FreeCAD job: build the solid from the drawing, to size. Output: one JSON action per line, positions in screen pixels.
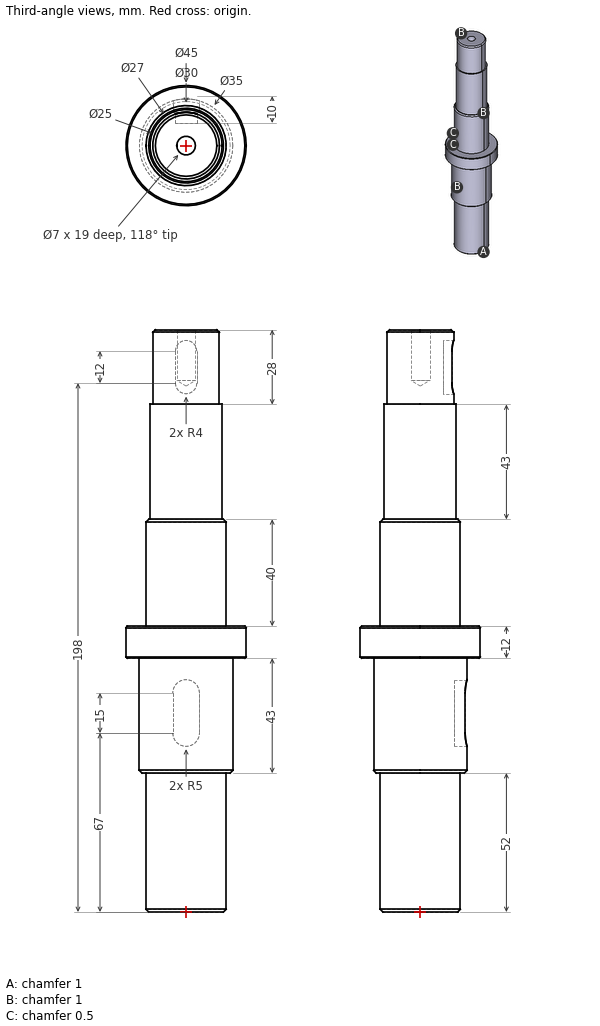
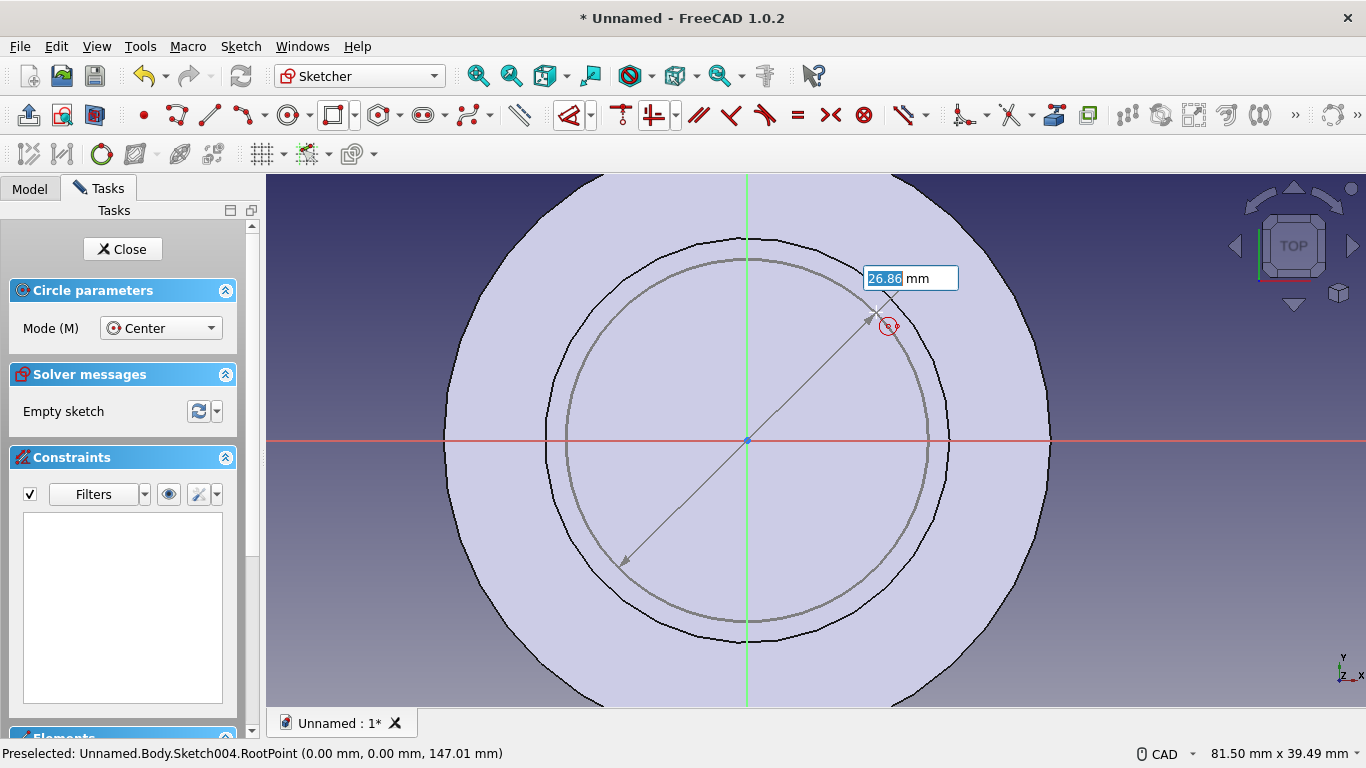
{"action": "type", "text": "27"}
{"action": "key", "text": "Return"}
{"action": "key", "text": "Escape"}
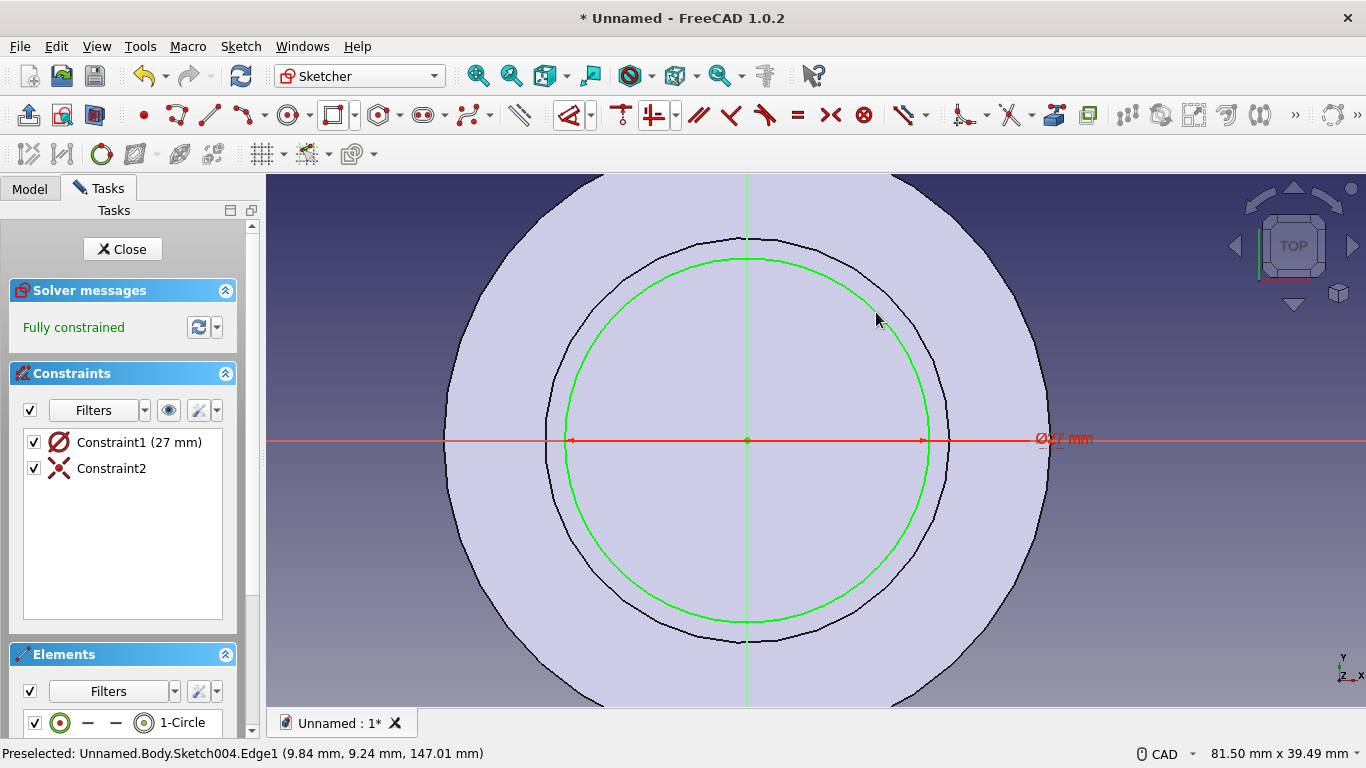
{"action": "left_click", "coordinate": [123, 249]}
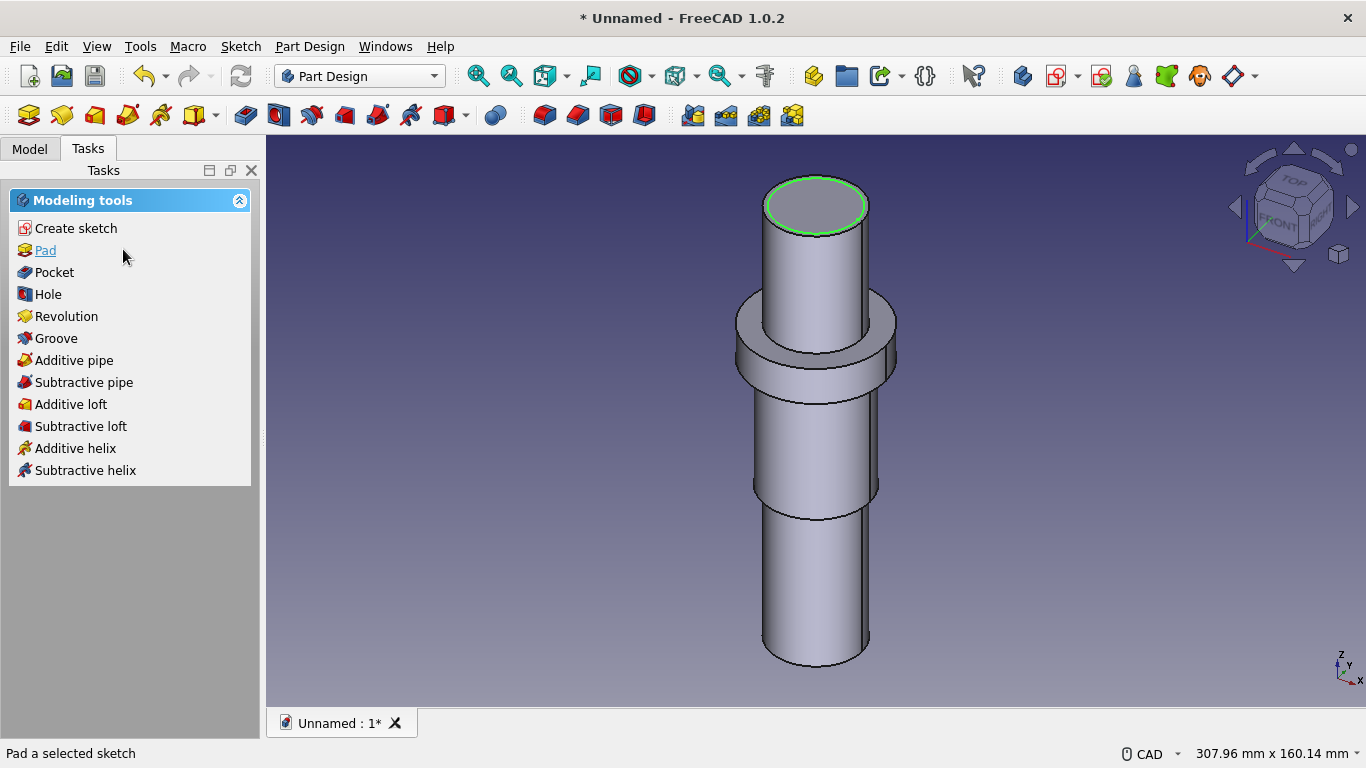
{"action": "left_click", "coordinate": [29, 116]}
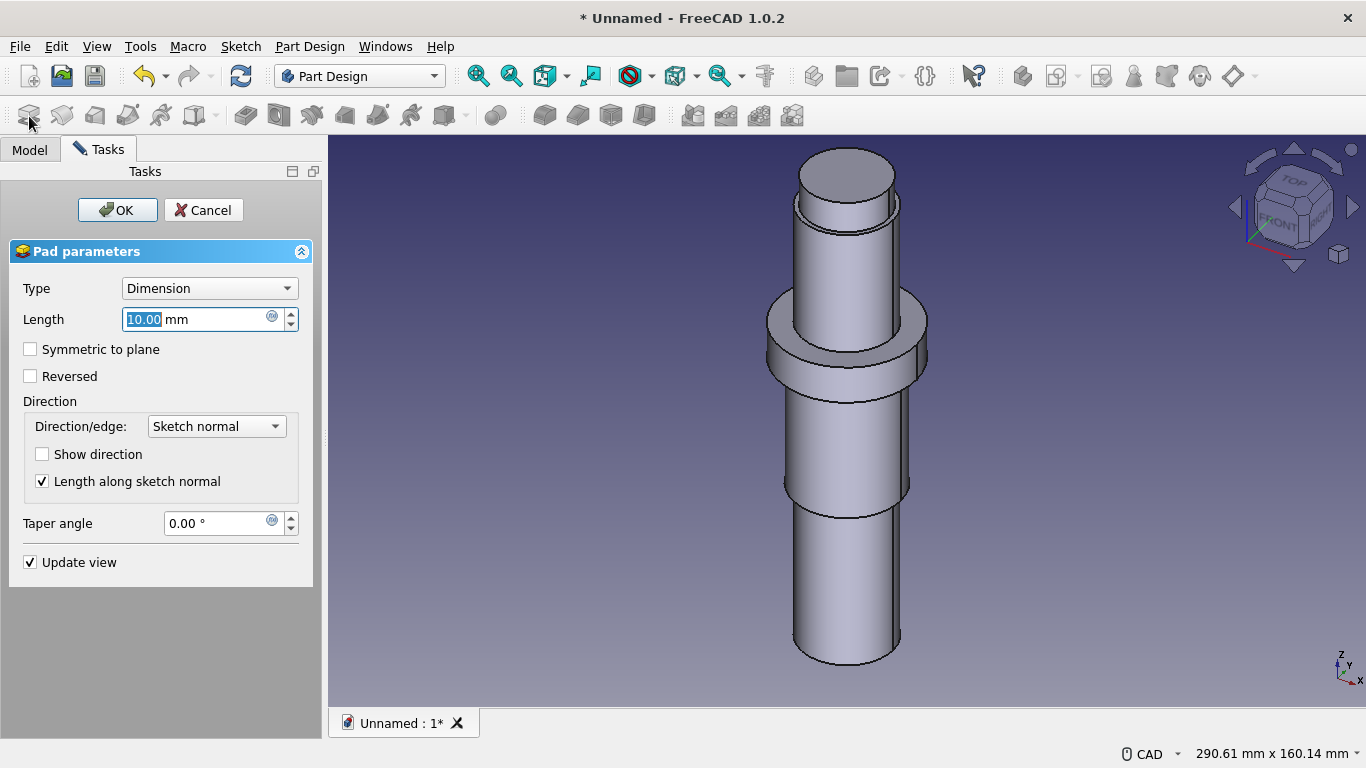
{"action": "type", "text": "43"}
{"action": "key", "text": "Tab"}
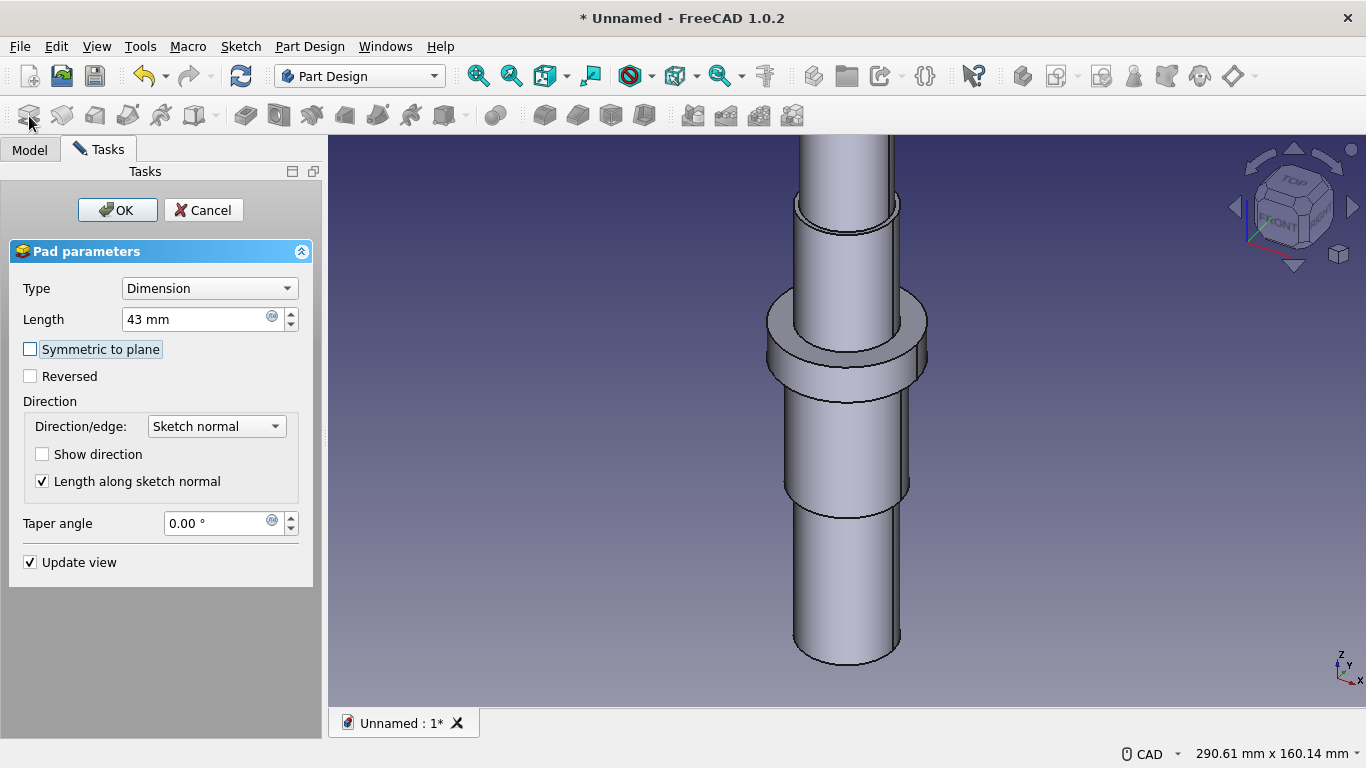
{"action": "left_click", "coordinate": [118, 210]}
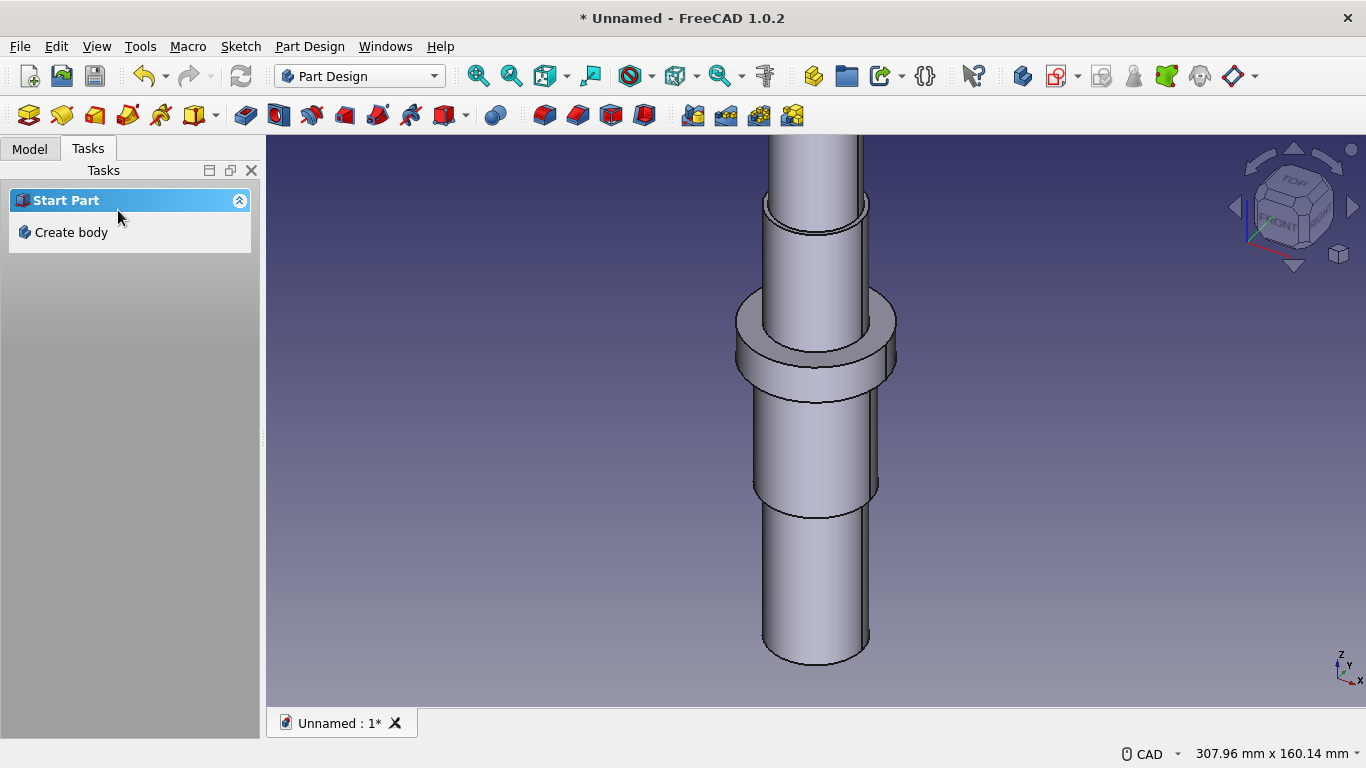
{"action": "key", "text": "v f"}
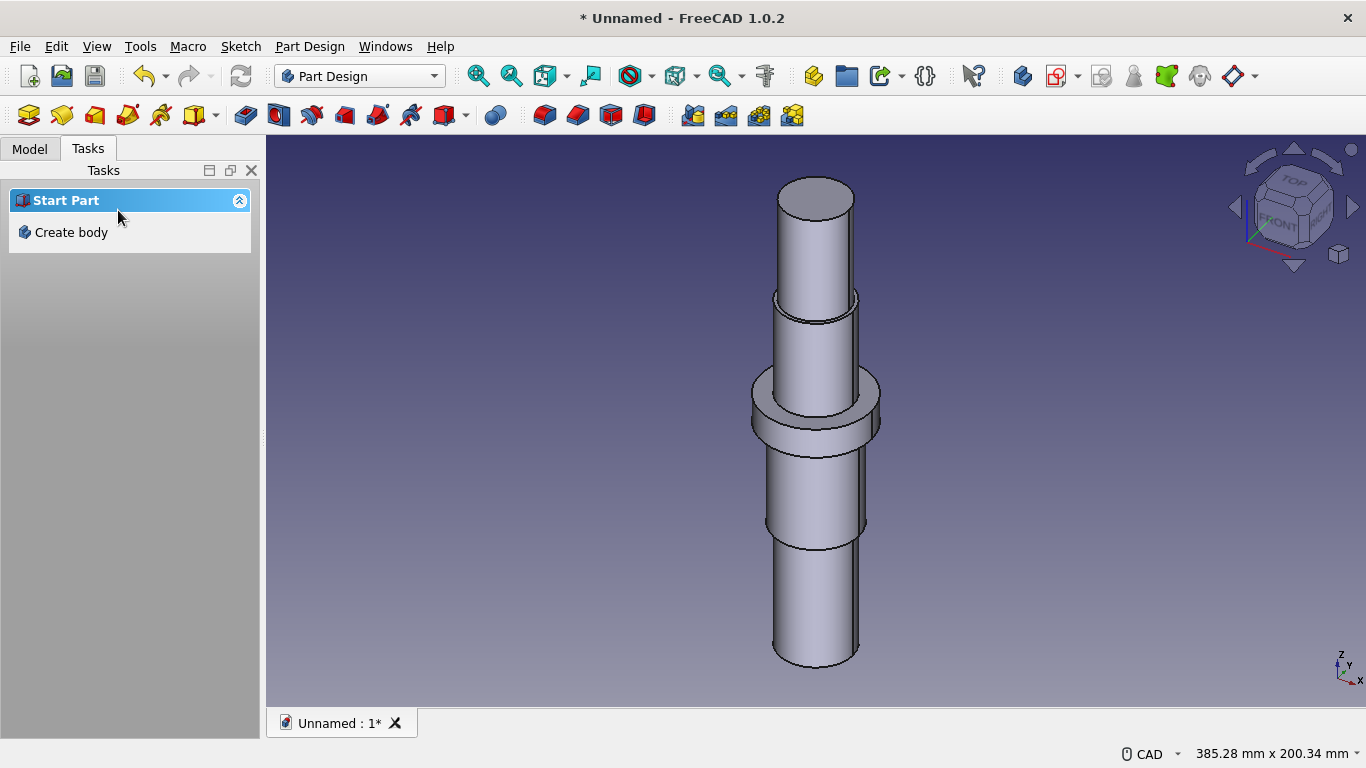
{"action": "left_click", "coordinate": [816, 198]}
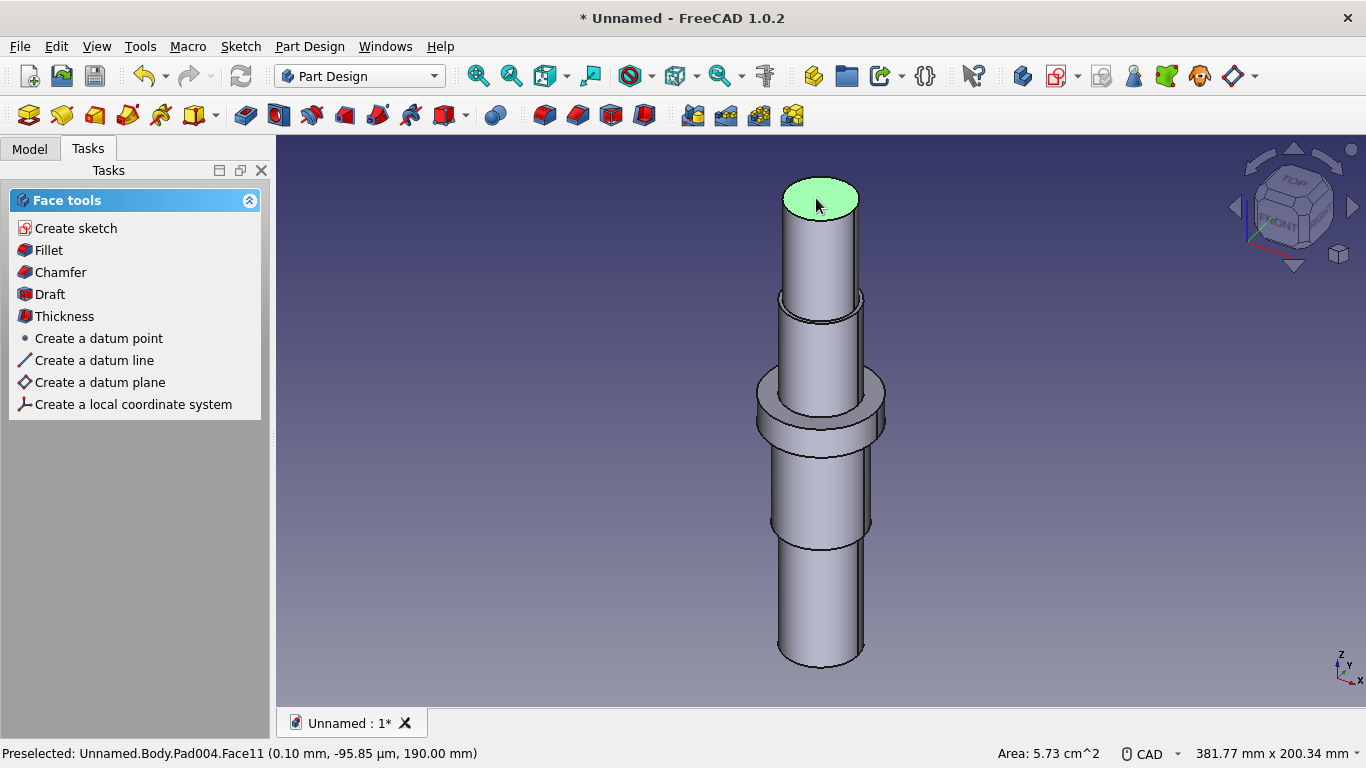
{"action": "left_click", "coordinate": [1056, 76]}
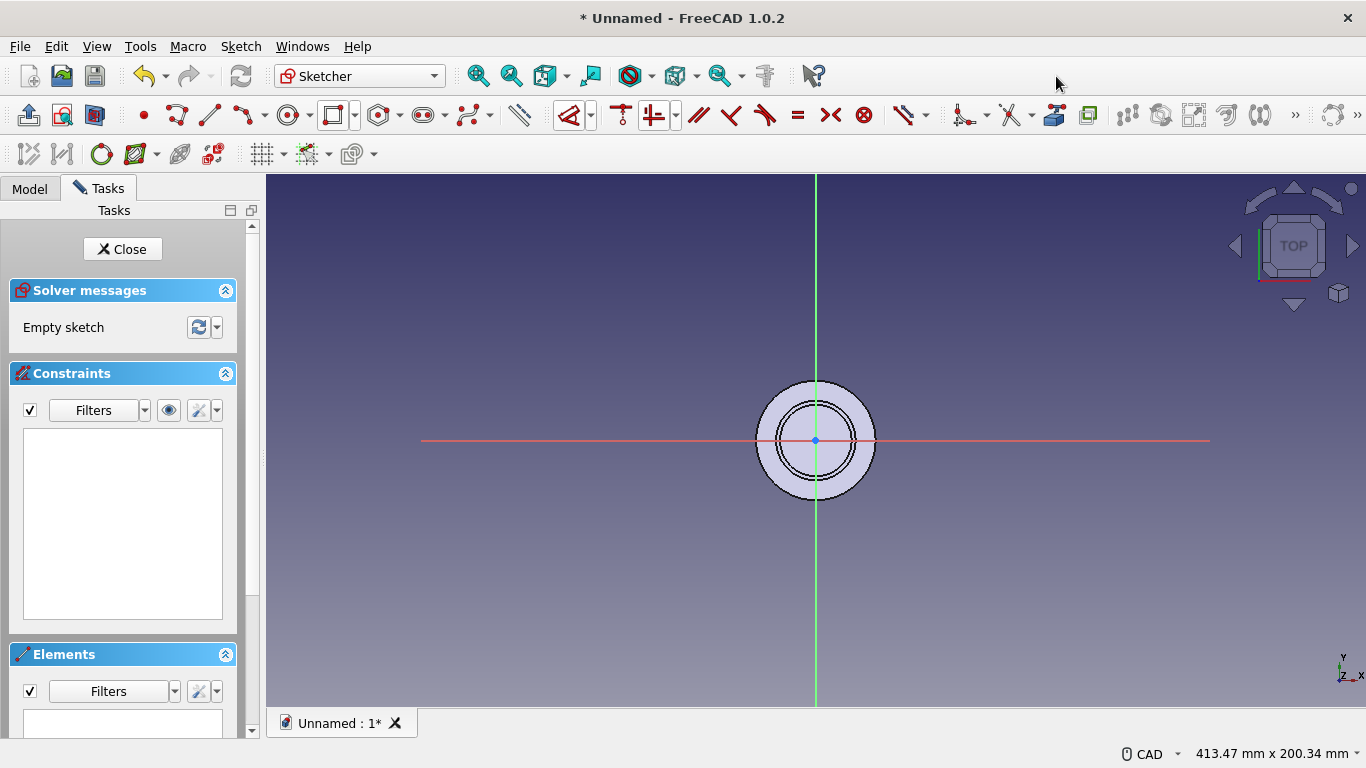
{"action": "scroll", "coordinate": [833, 440], "scroll_direction": "up", "scroll_amount": 8}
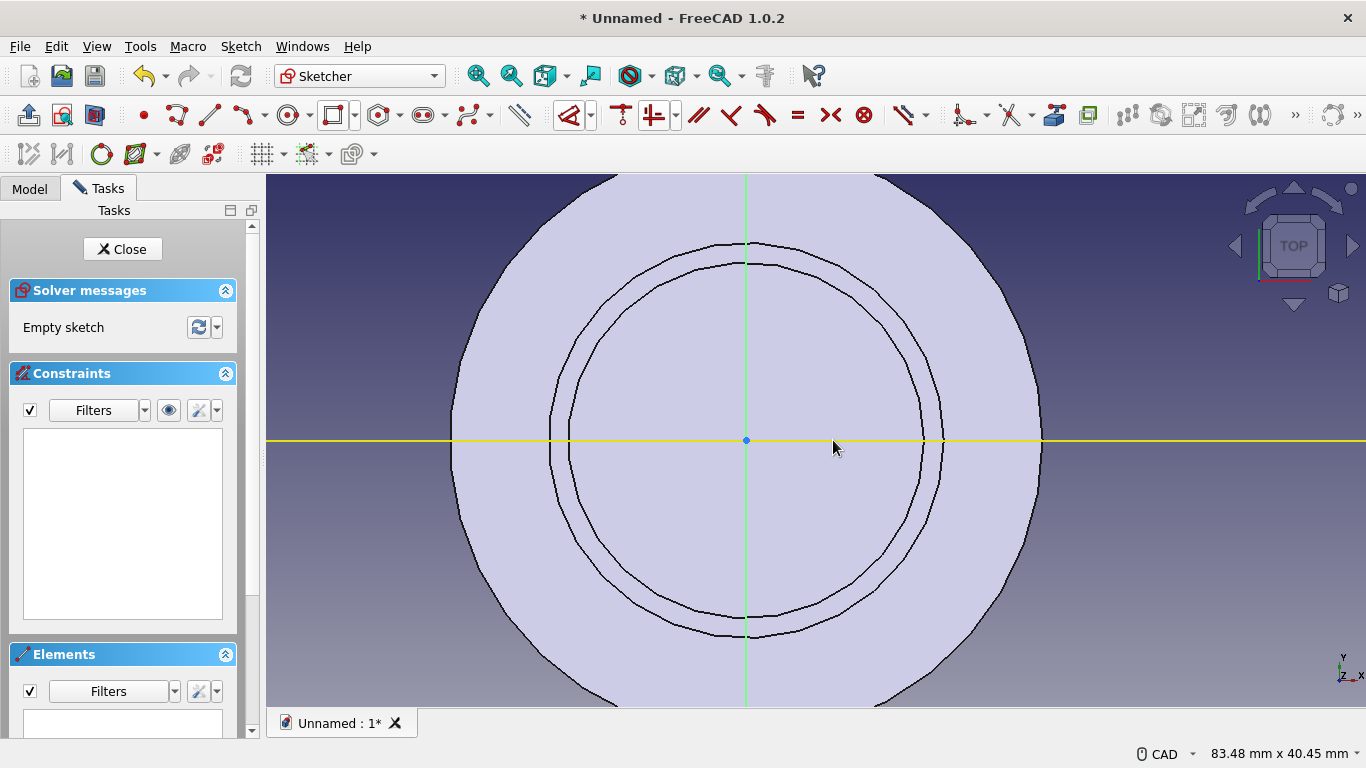
{"action": "left_click", "coordinate": [288, 116]}